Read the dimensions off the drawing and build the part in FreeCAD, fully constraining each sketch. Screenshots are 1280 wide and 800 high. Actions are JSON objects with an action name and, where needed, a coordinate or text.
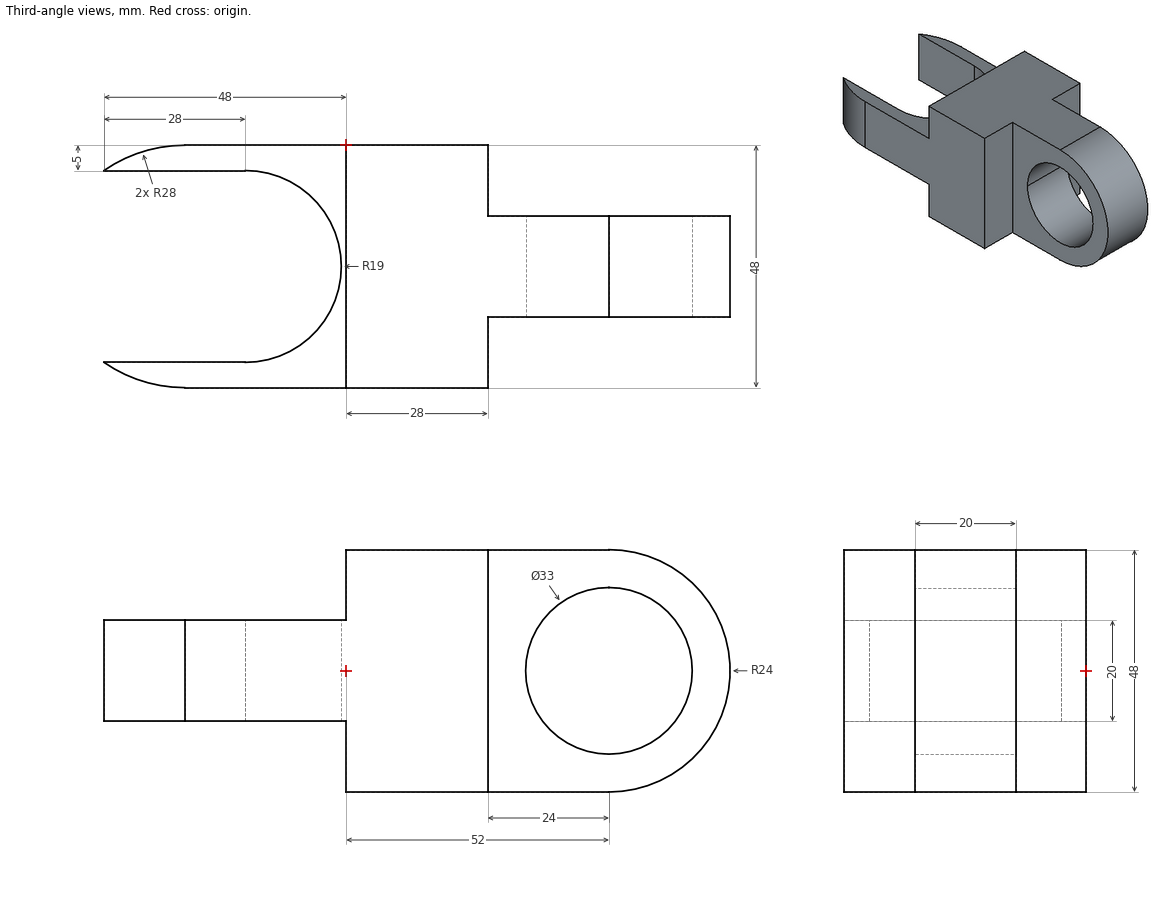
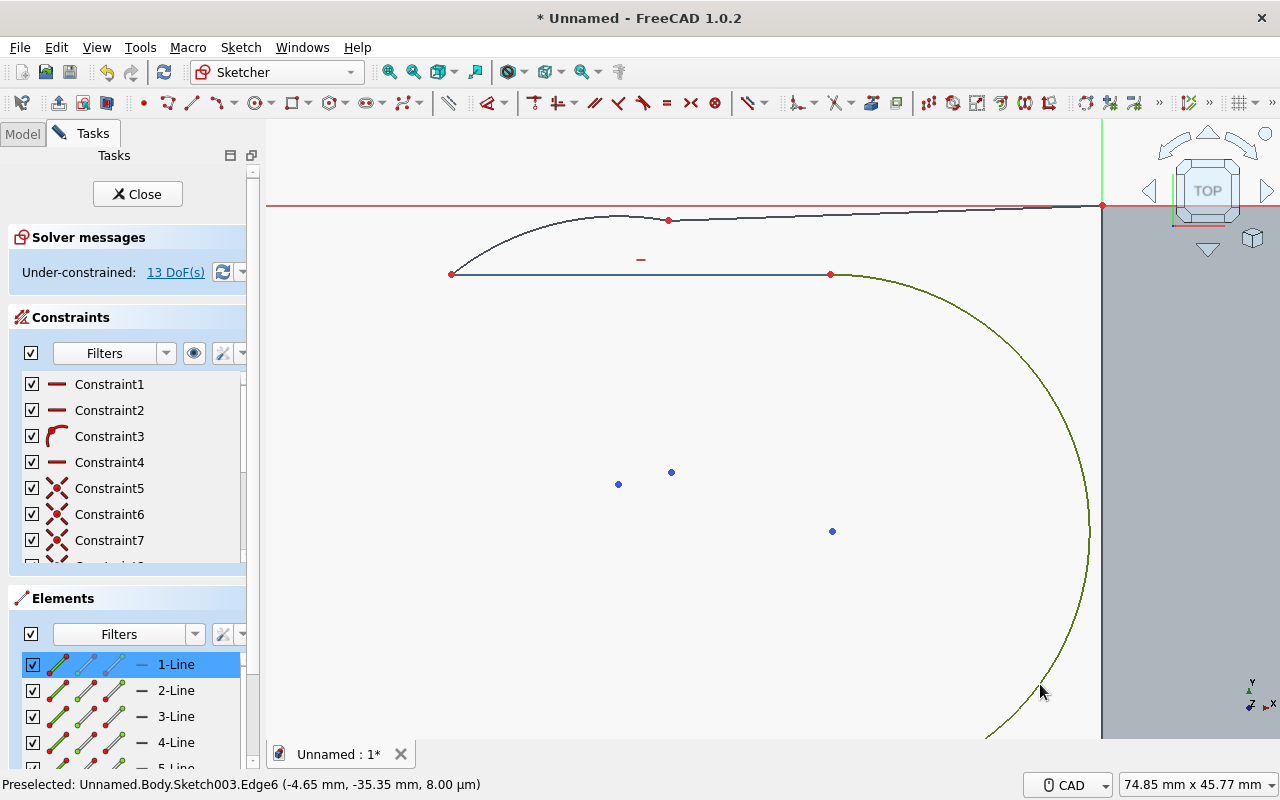
{"action": "left_click", "coordinate": [644, 104]}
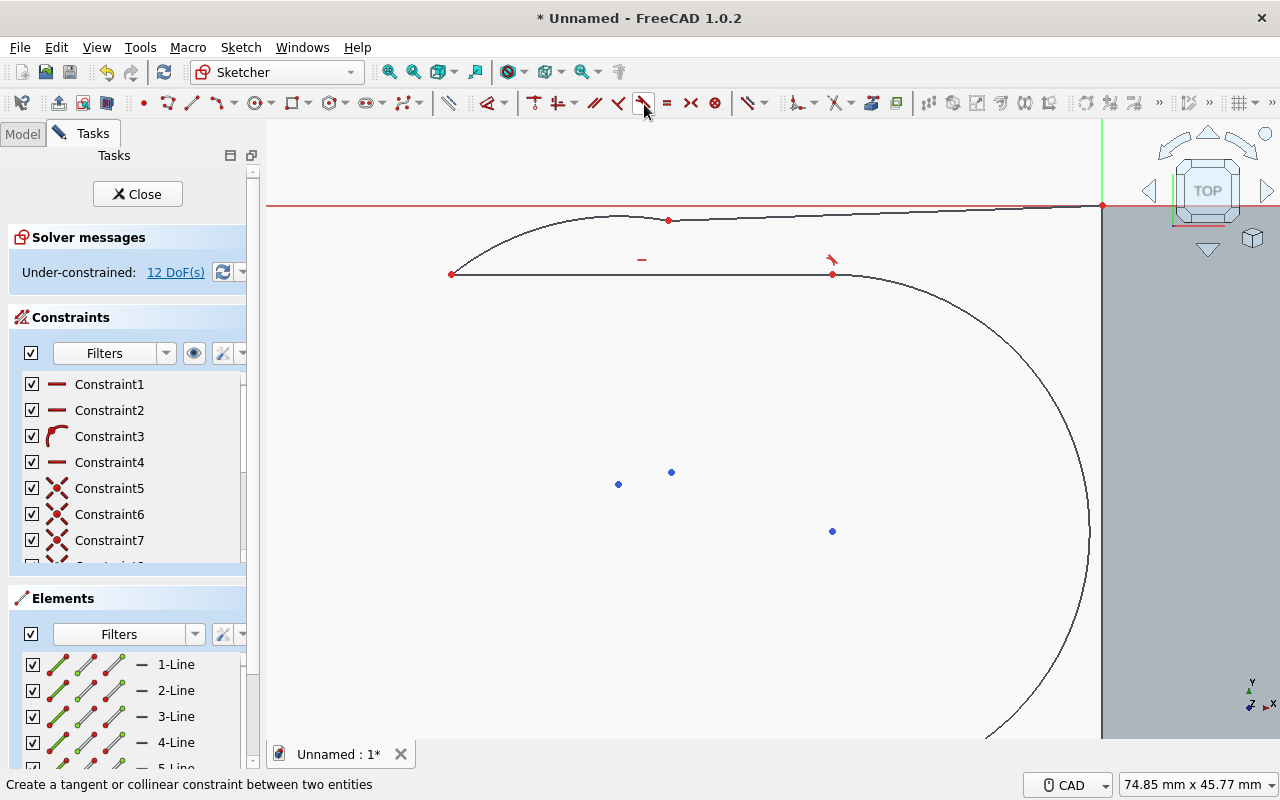
{"action": "scroll", "coordinate": [556, 222], "scroll_direction": "down", "scroll_amount": 2}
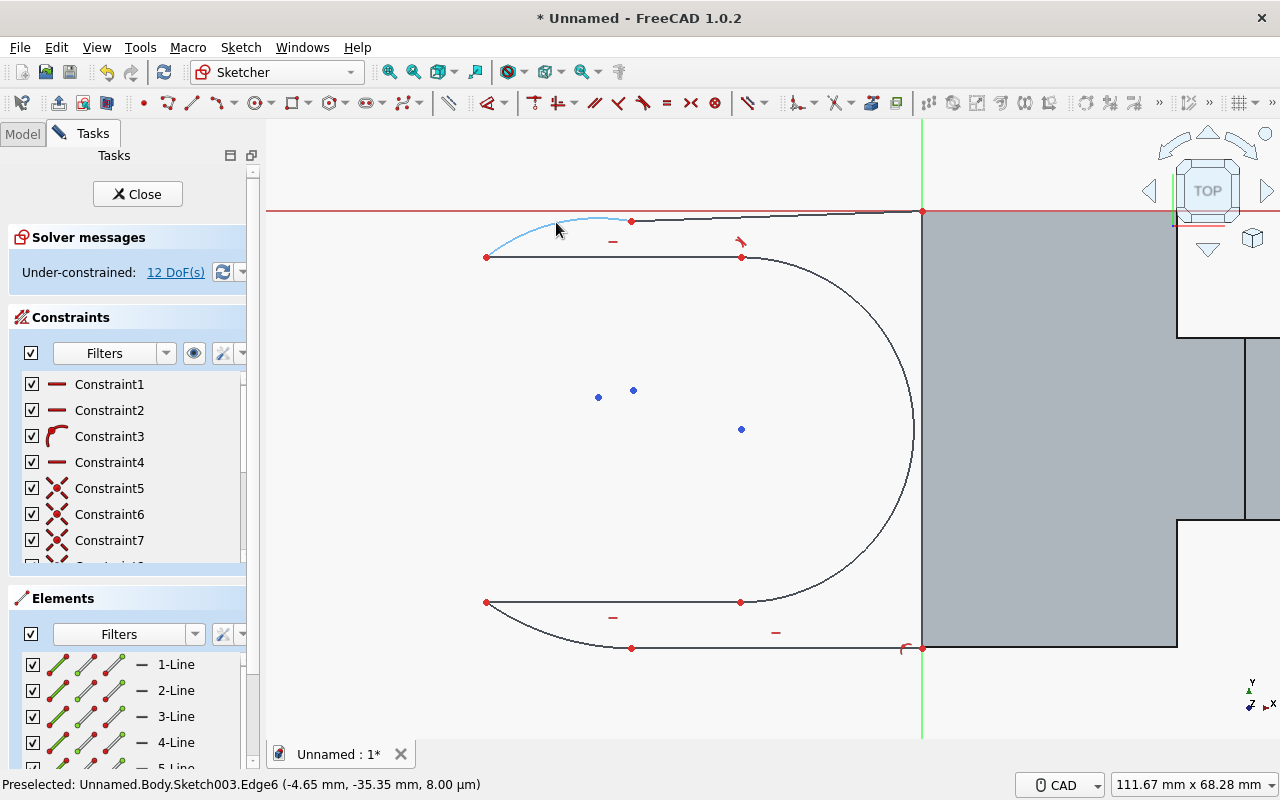
{"action": "left_click", "coordinate": [664, 602]}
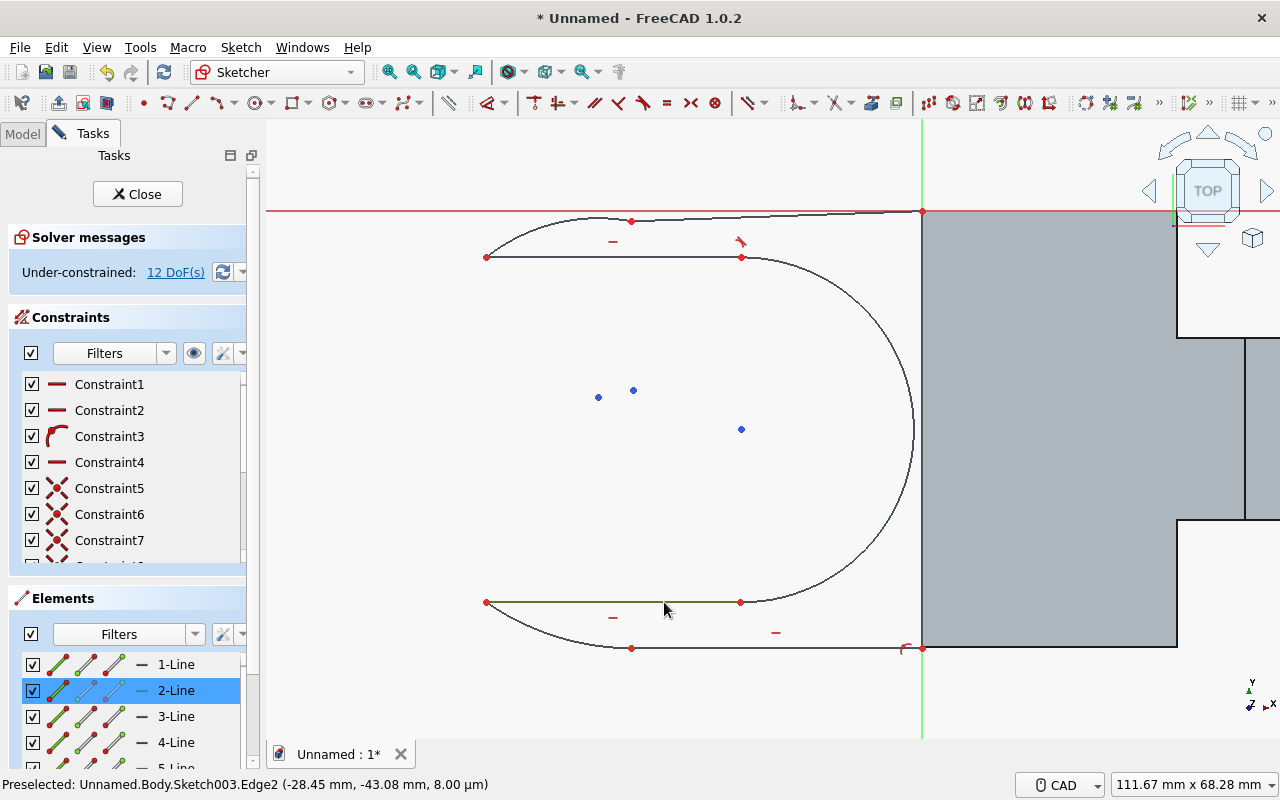
{"action": "left_click", "coordinate": [880, 532]}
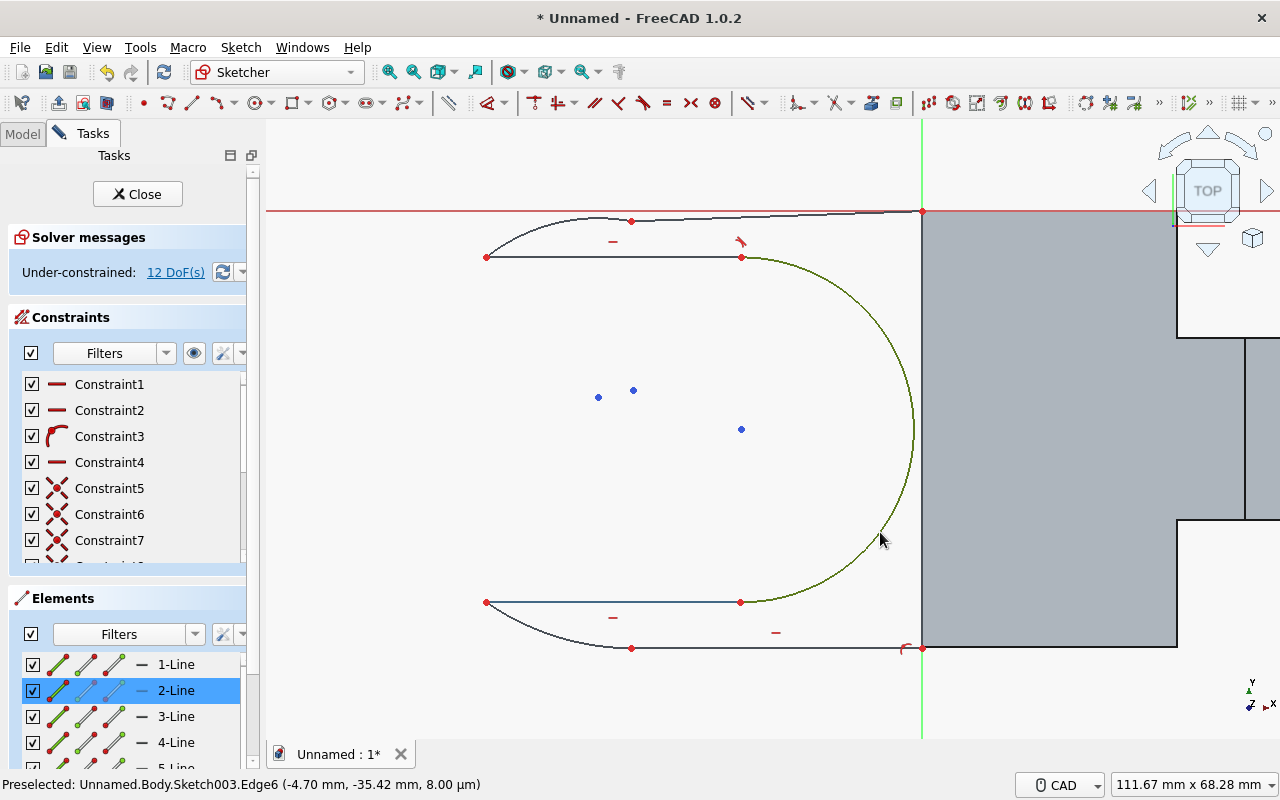
{"action": "left_click", "coordinate": [644, 104]}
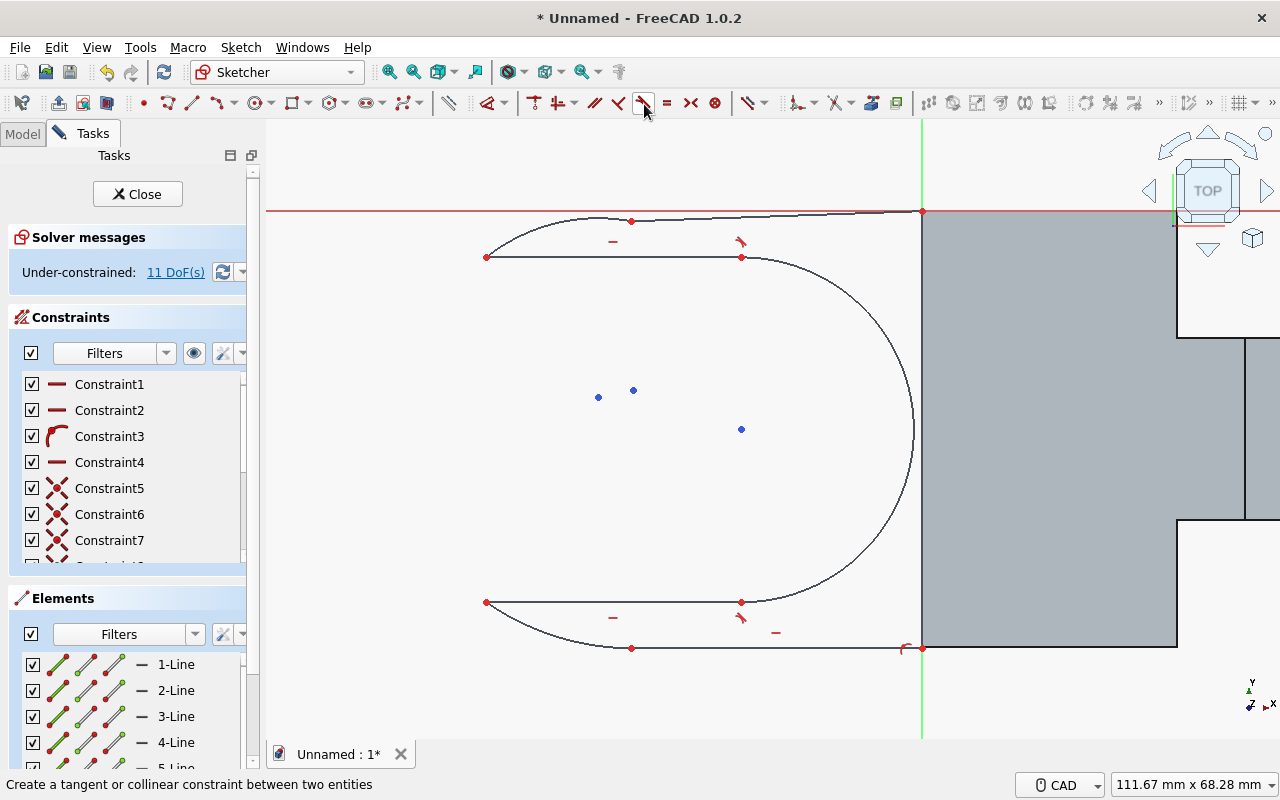
{"action": "left_click", "coordinate": [719, 648]}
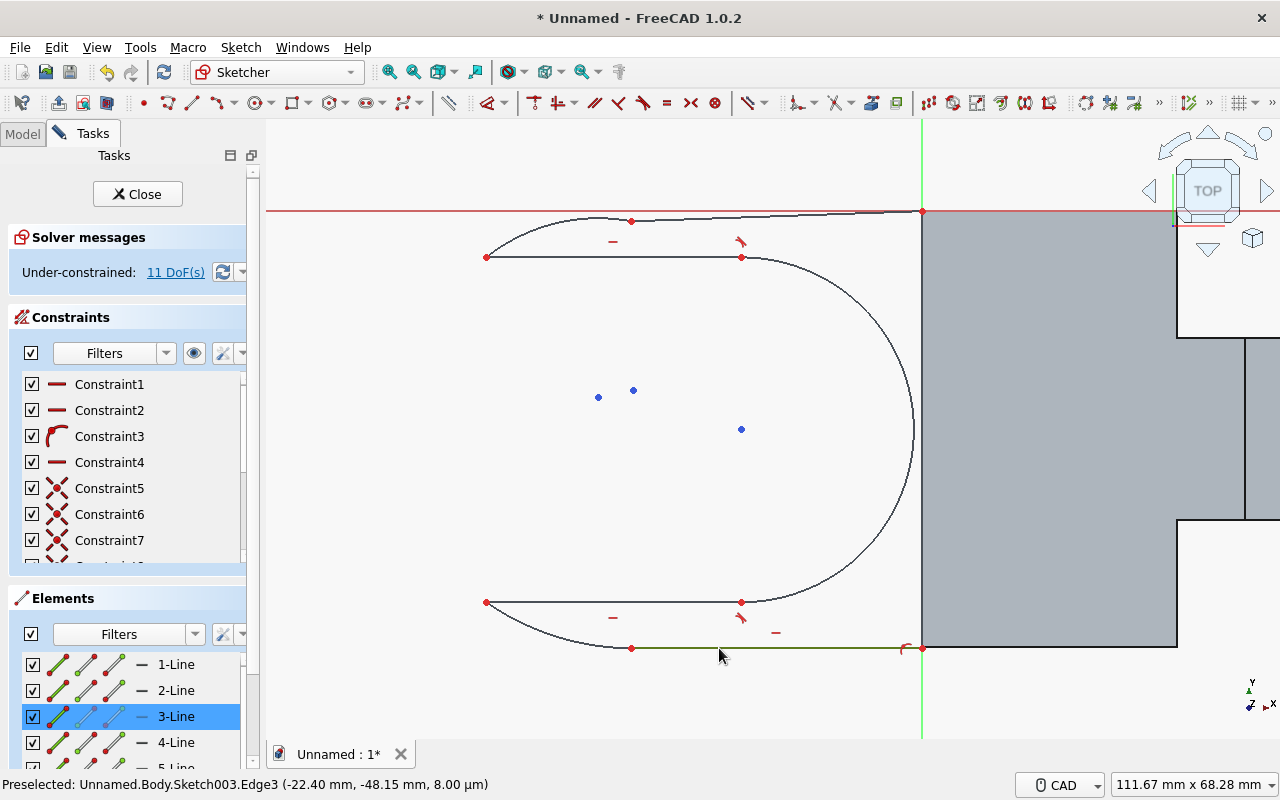
{"action": "left_click", "coordinate": [527, 625]}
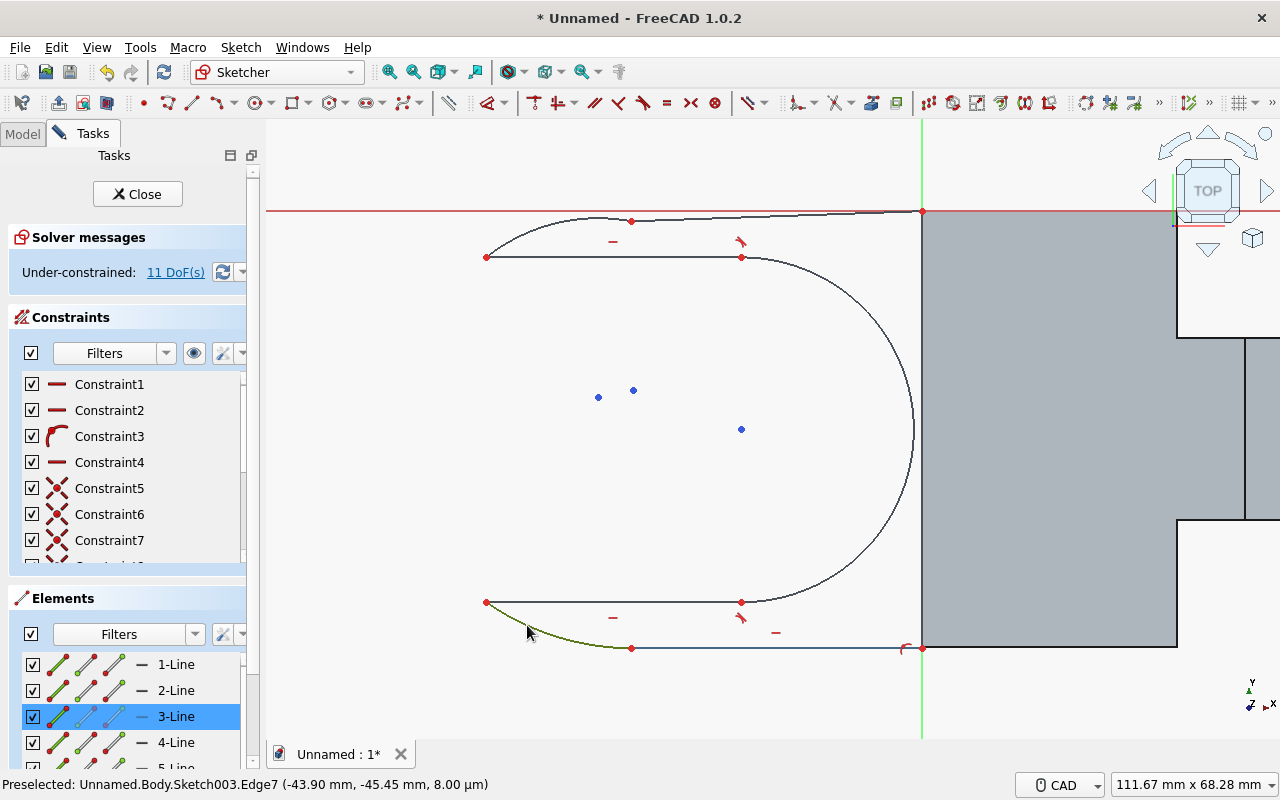
{"action": "left_click", "coordinate": [644, 104]}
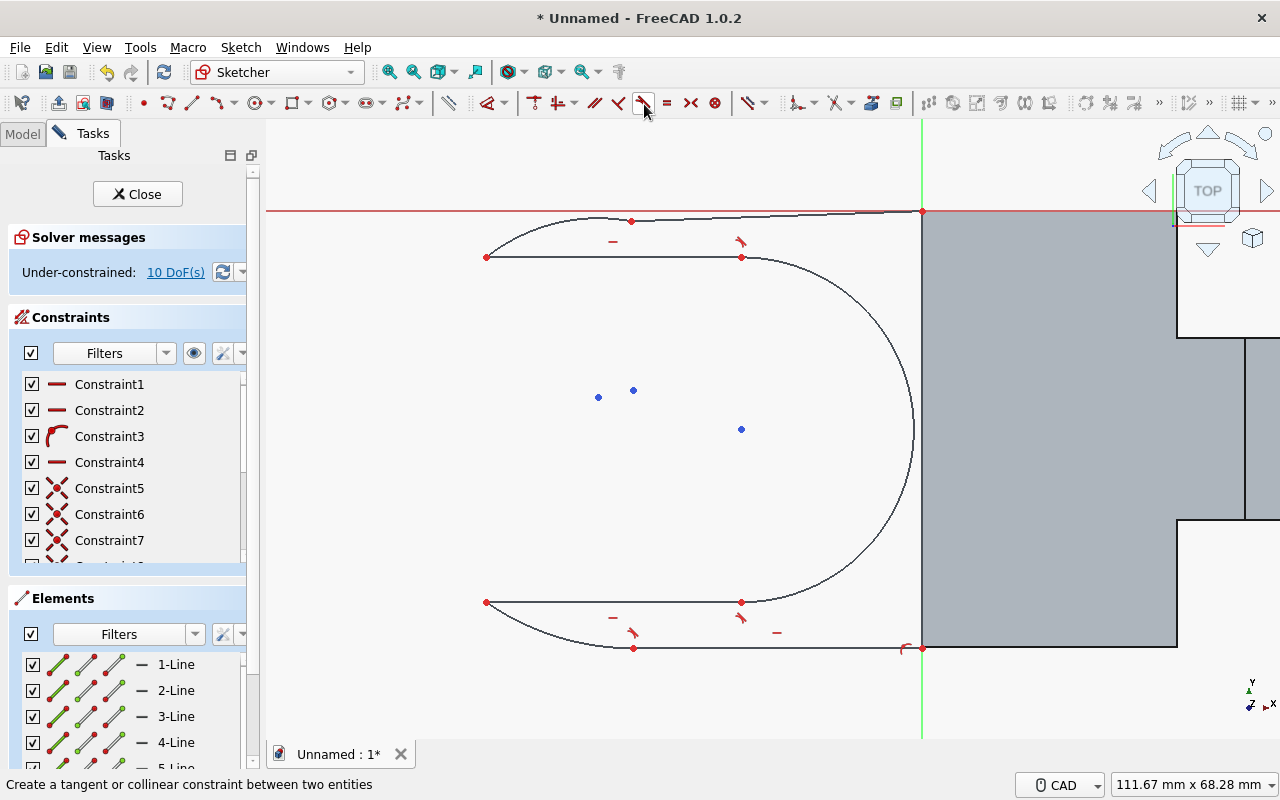
{"action": "left_click", "coordinate": [835, 214]}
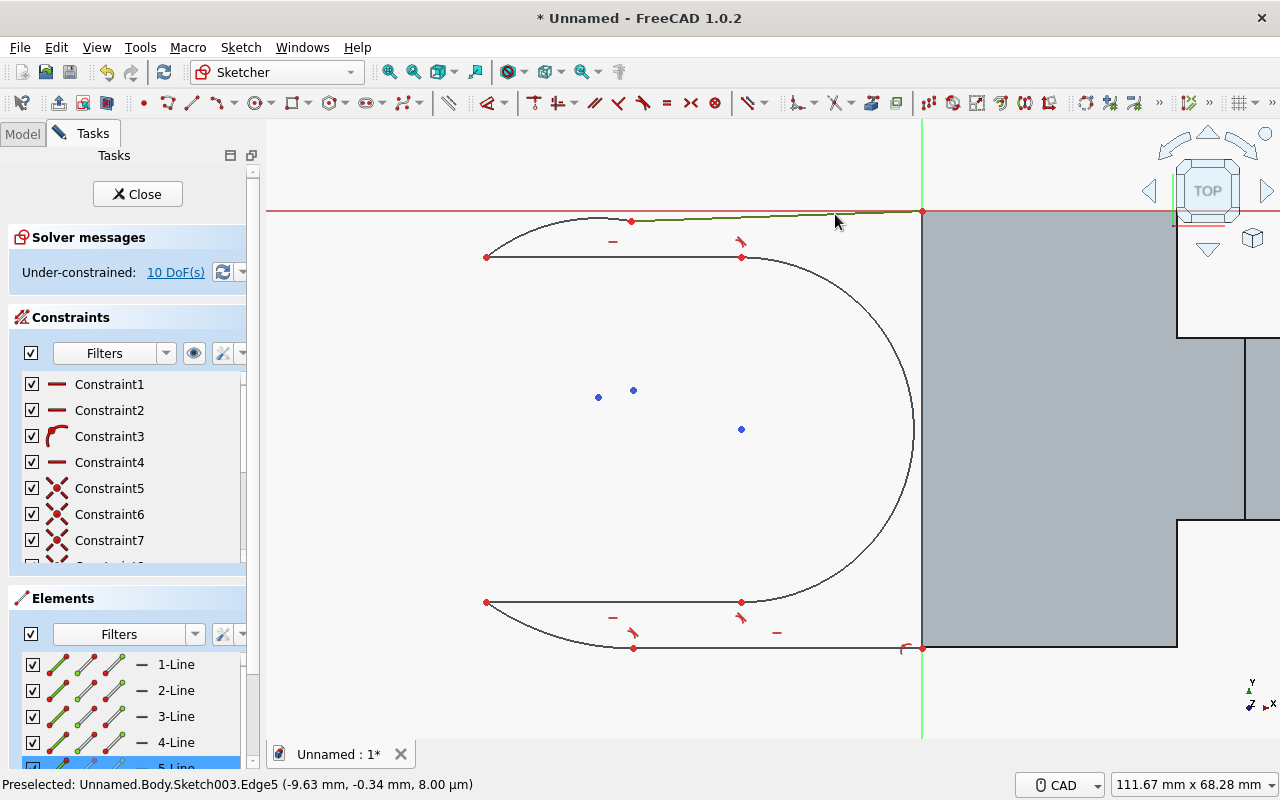
{"action": "left_click", "coordinate": [526, 233]}